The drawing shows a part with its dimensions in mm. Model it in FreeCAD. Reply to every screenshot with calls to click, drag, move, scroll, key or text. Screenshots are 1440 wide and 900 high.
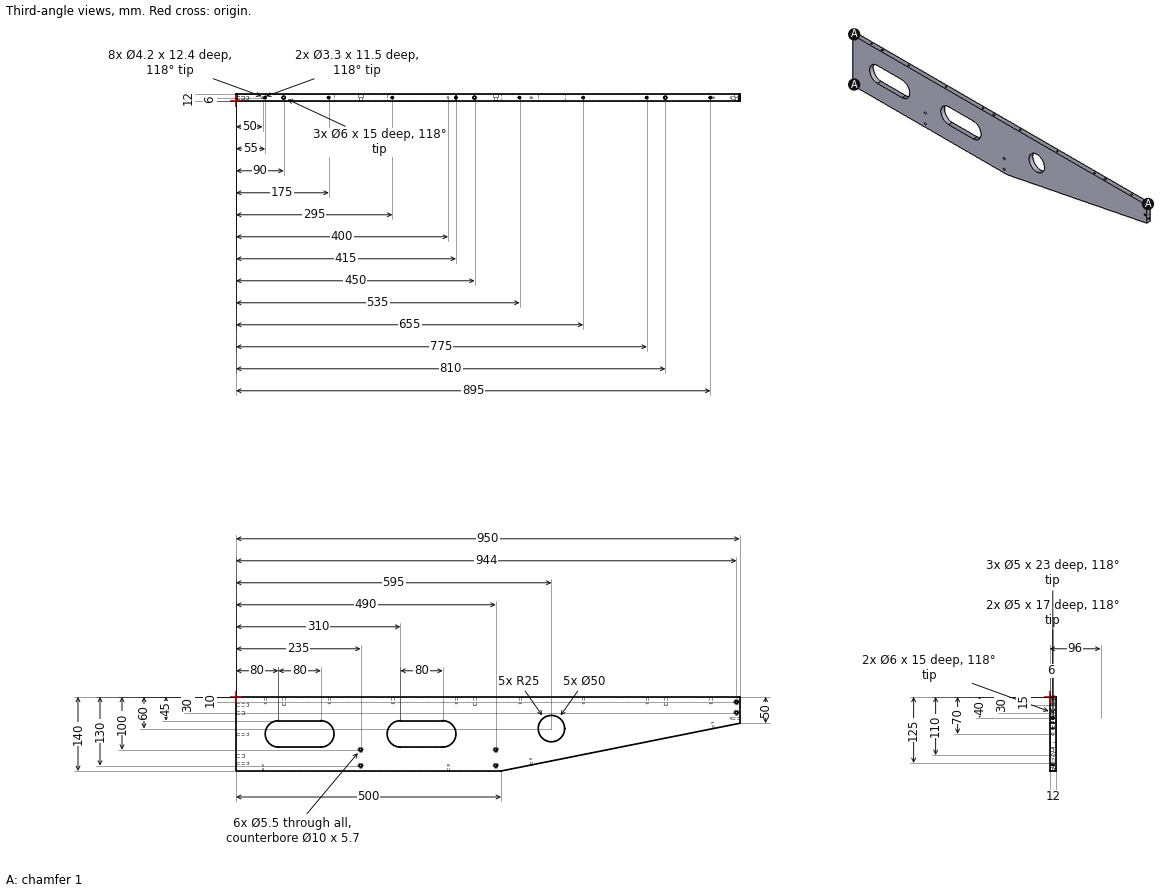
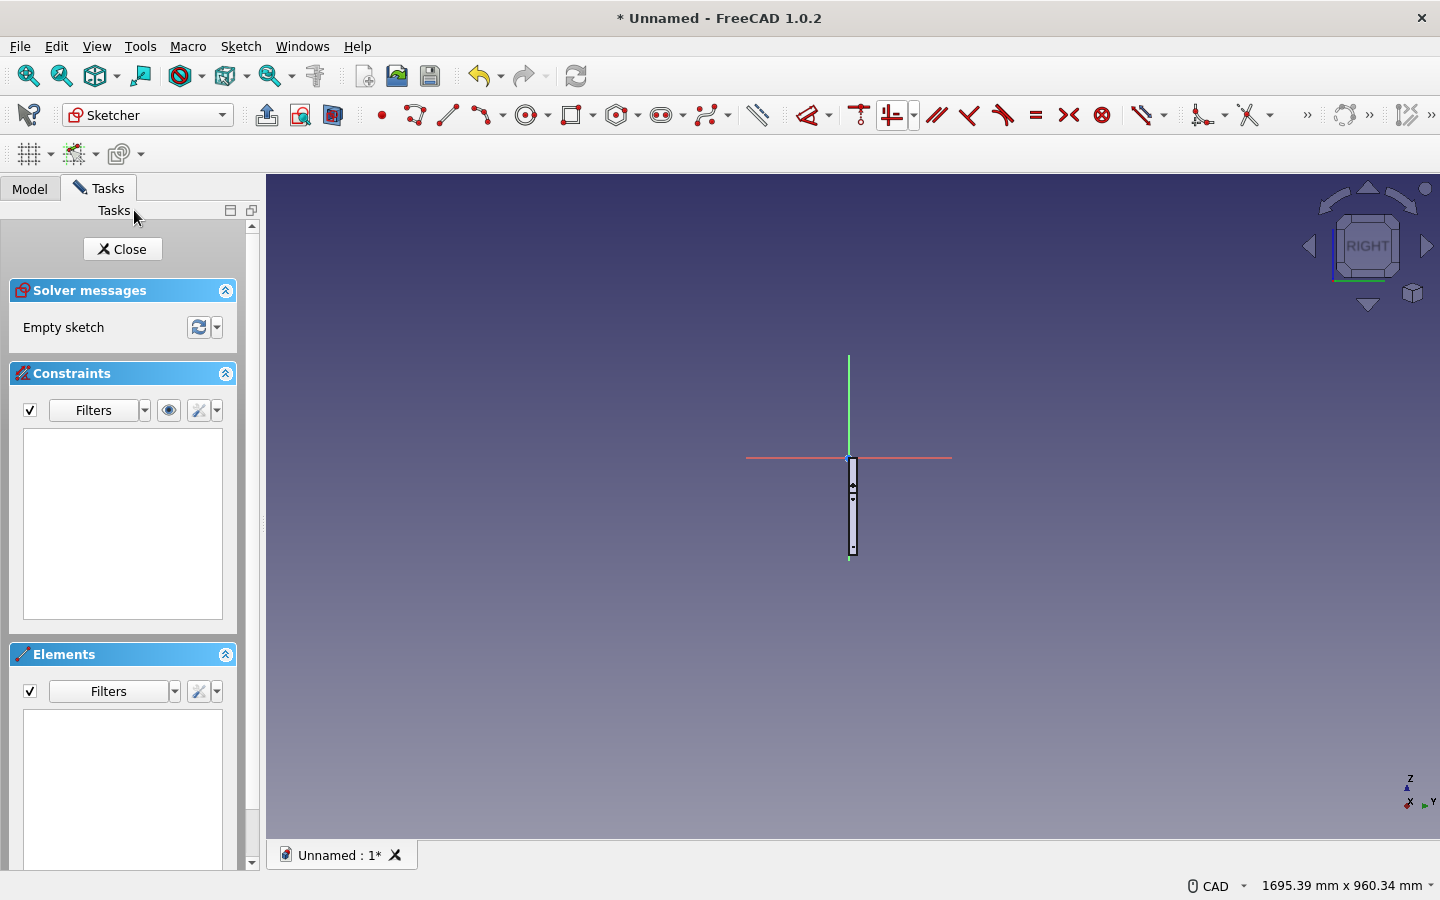
click(333, 116)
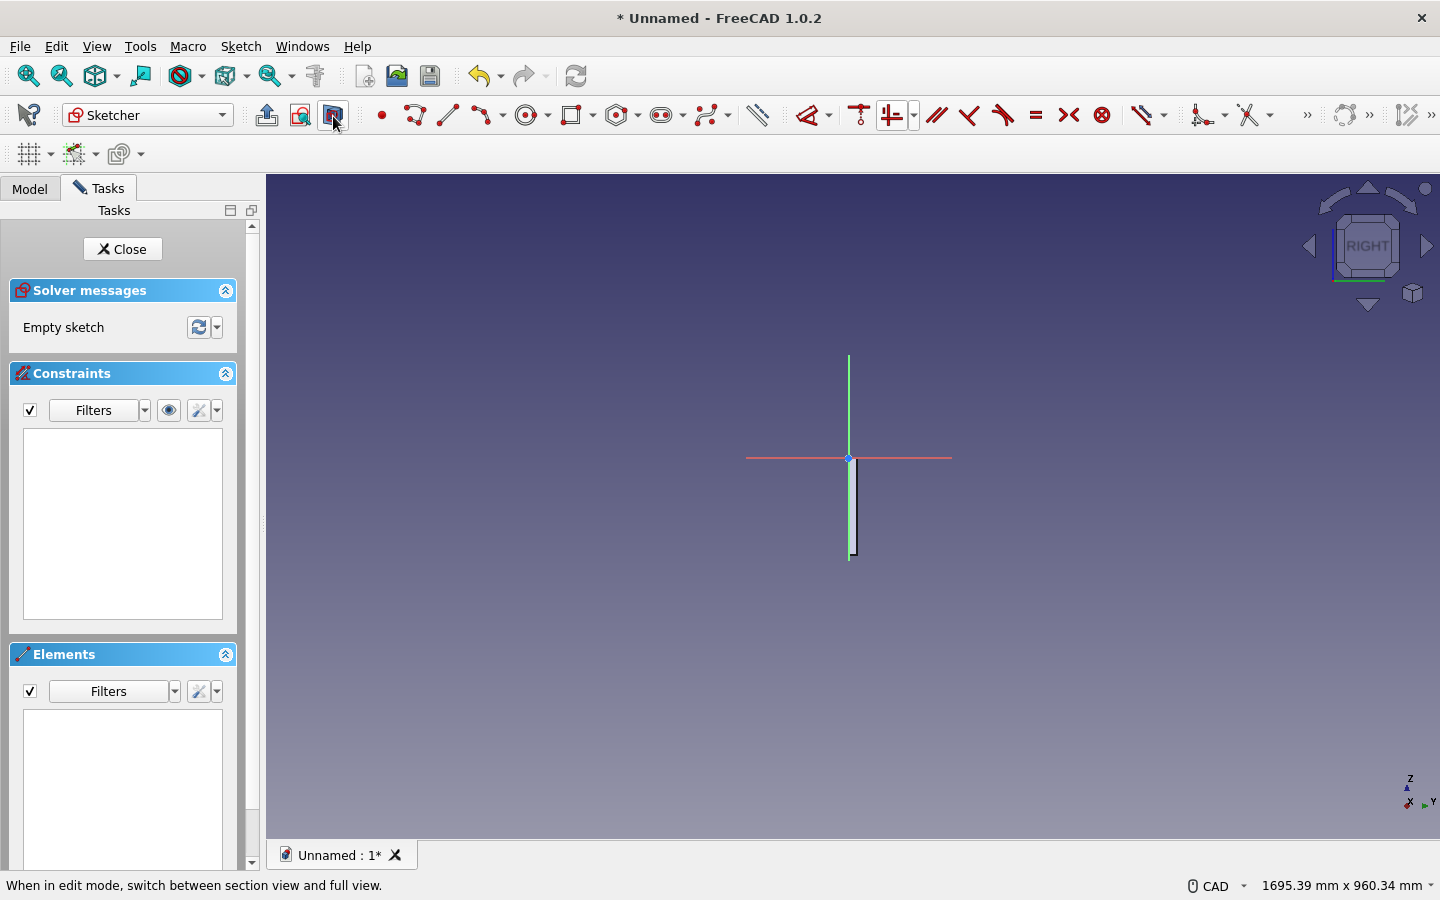
scroll(869, 501, up, 8)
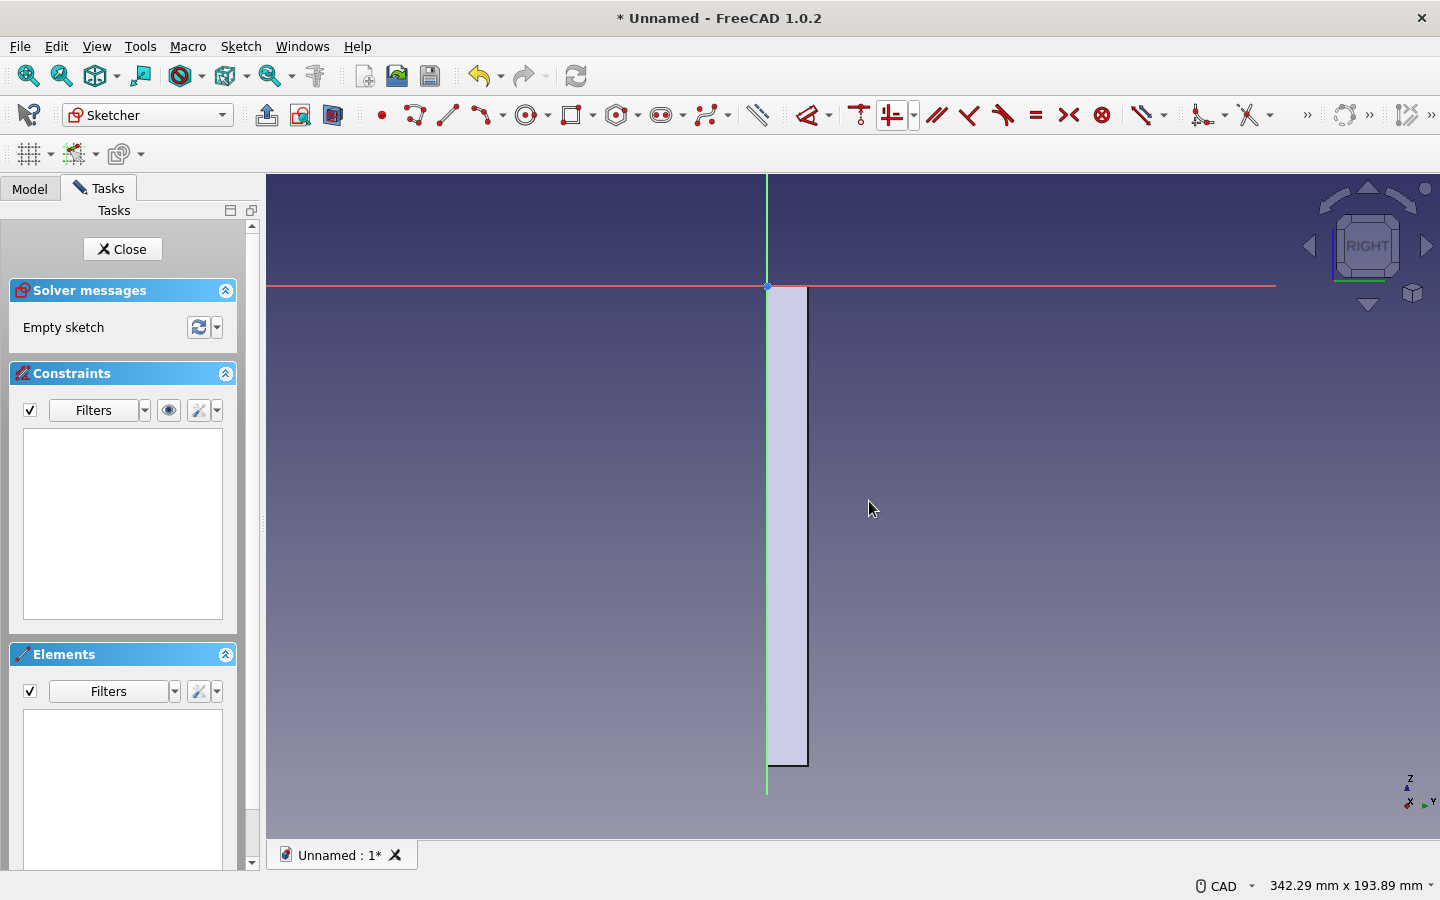
click(526, 116)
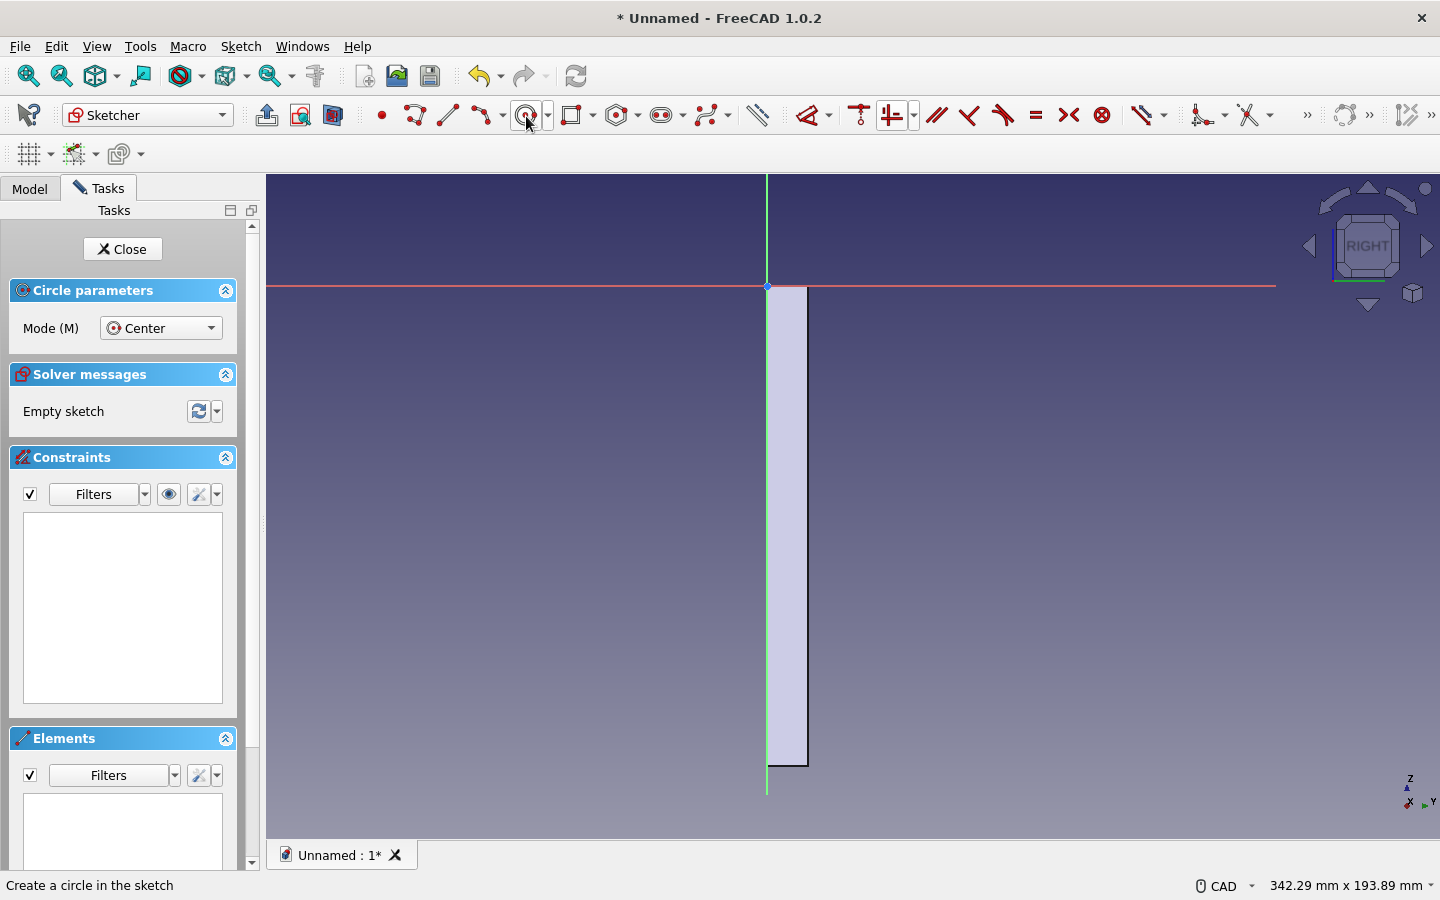
scroll(788, 338, up, 5)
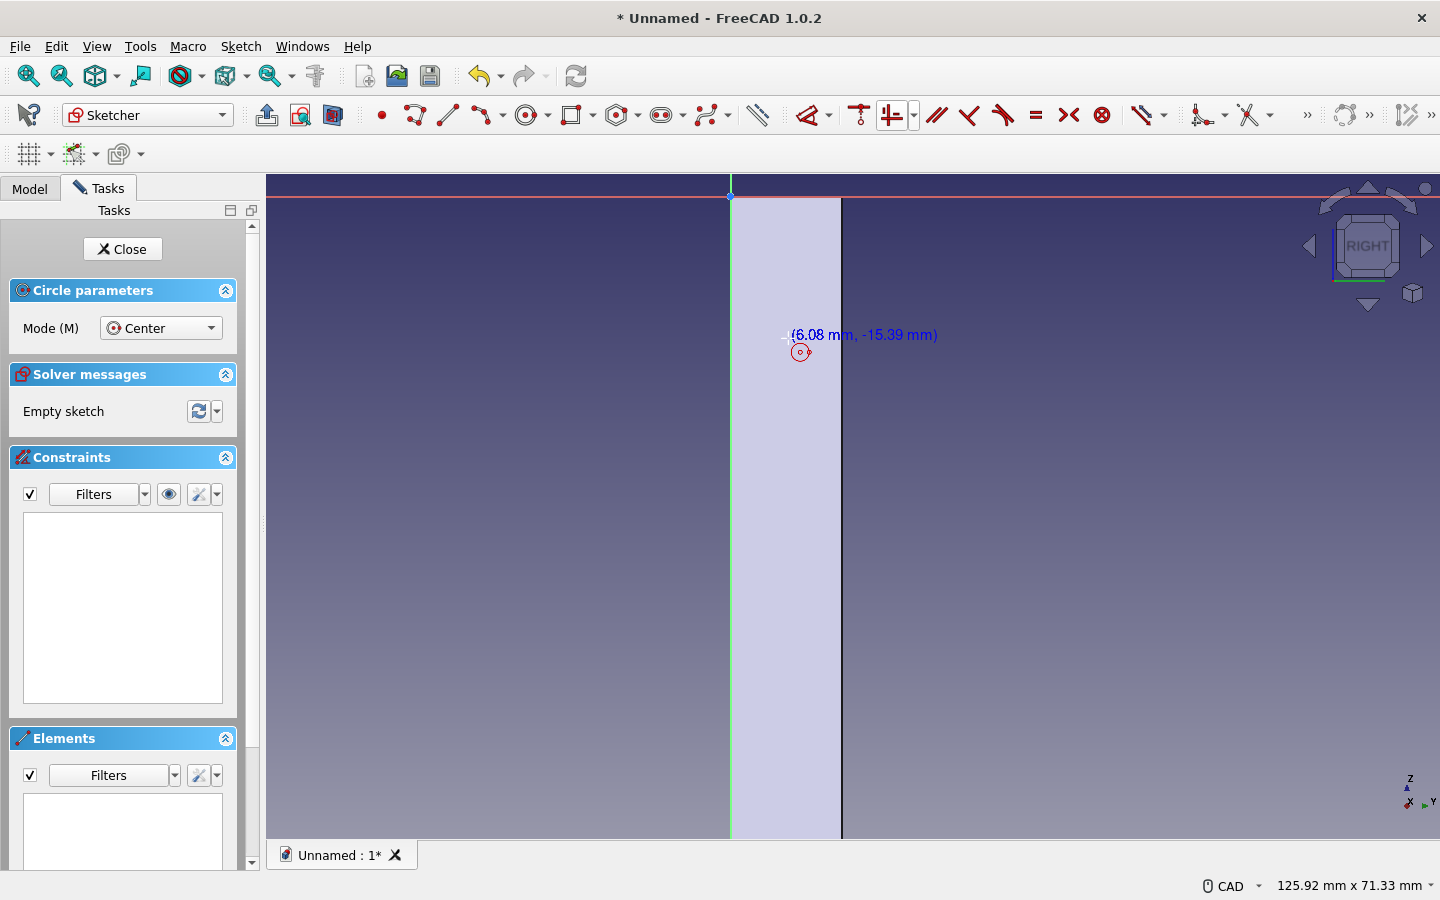
click(786, 337)
move(803, 320)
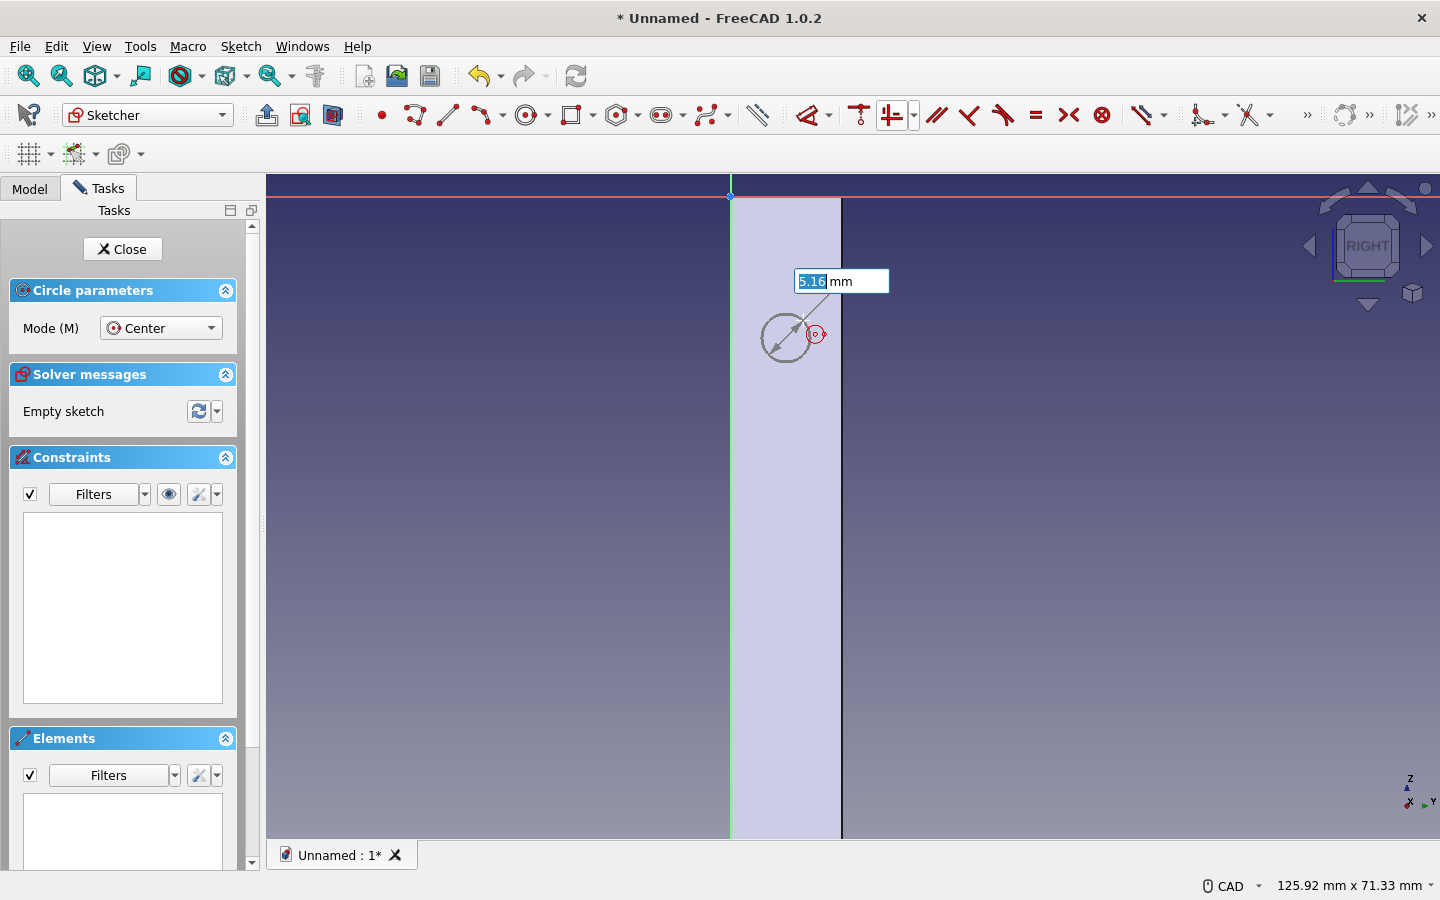
text(5)
key(Return)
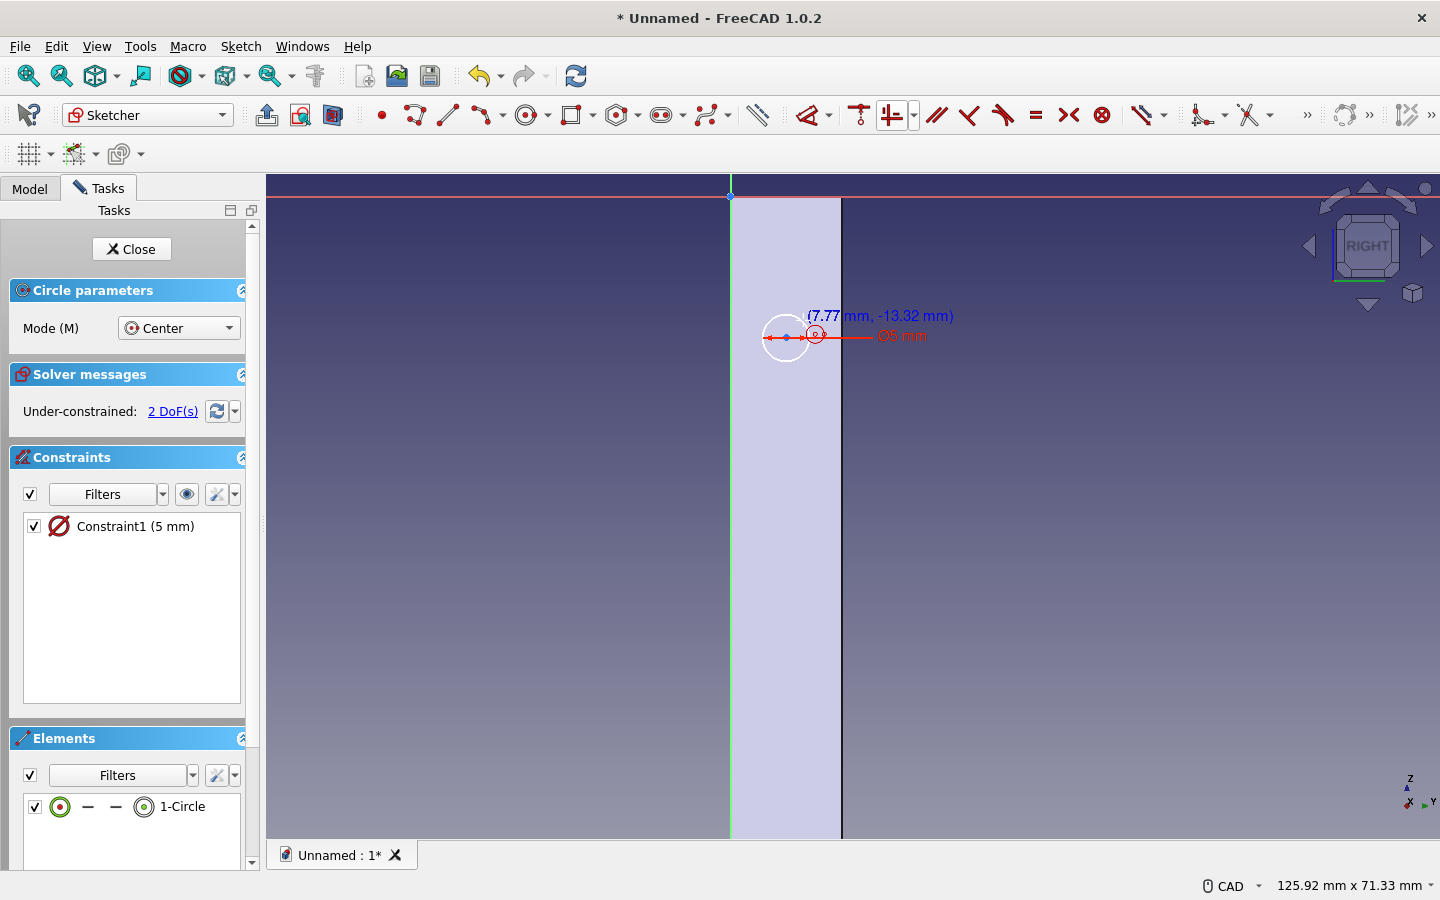
scroll(793, 341, down, 5)